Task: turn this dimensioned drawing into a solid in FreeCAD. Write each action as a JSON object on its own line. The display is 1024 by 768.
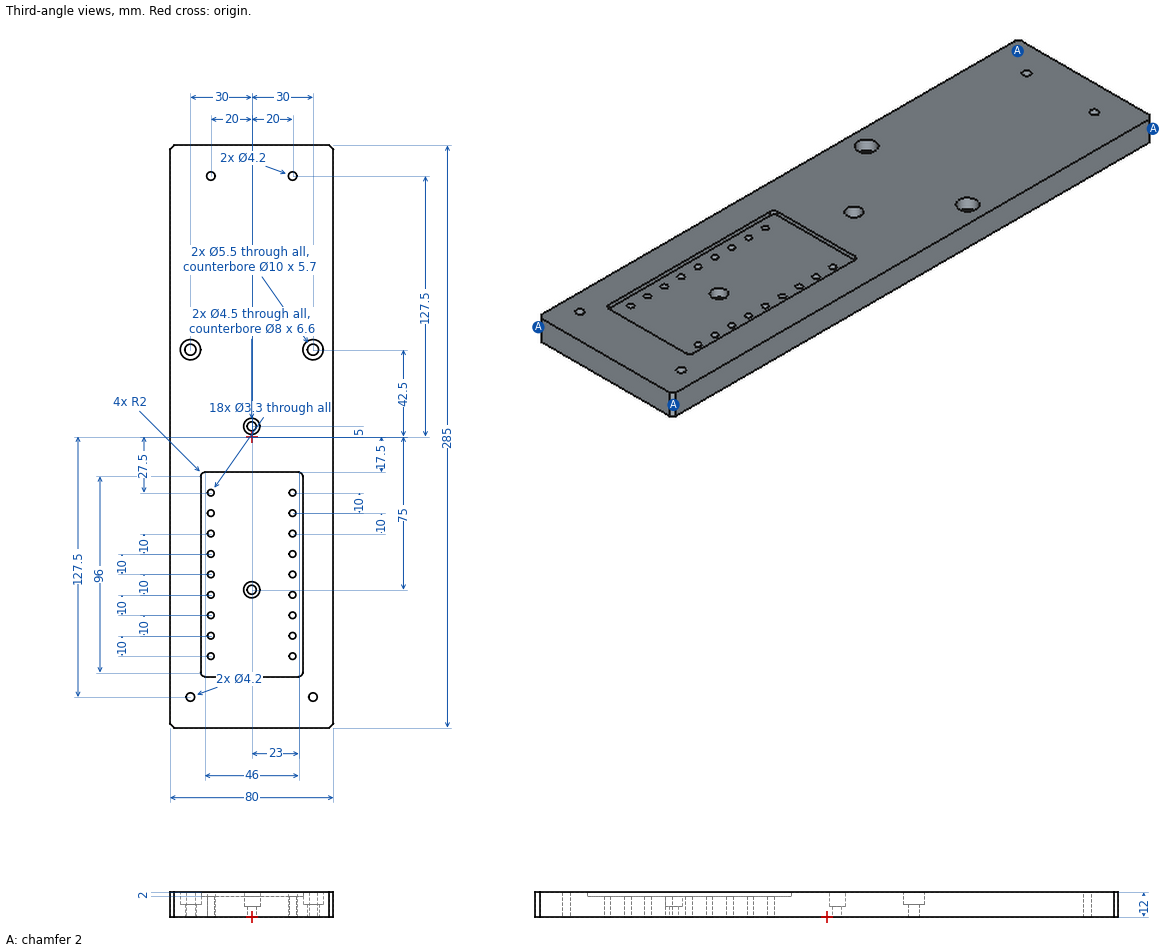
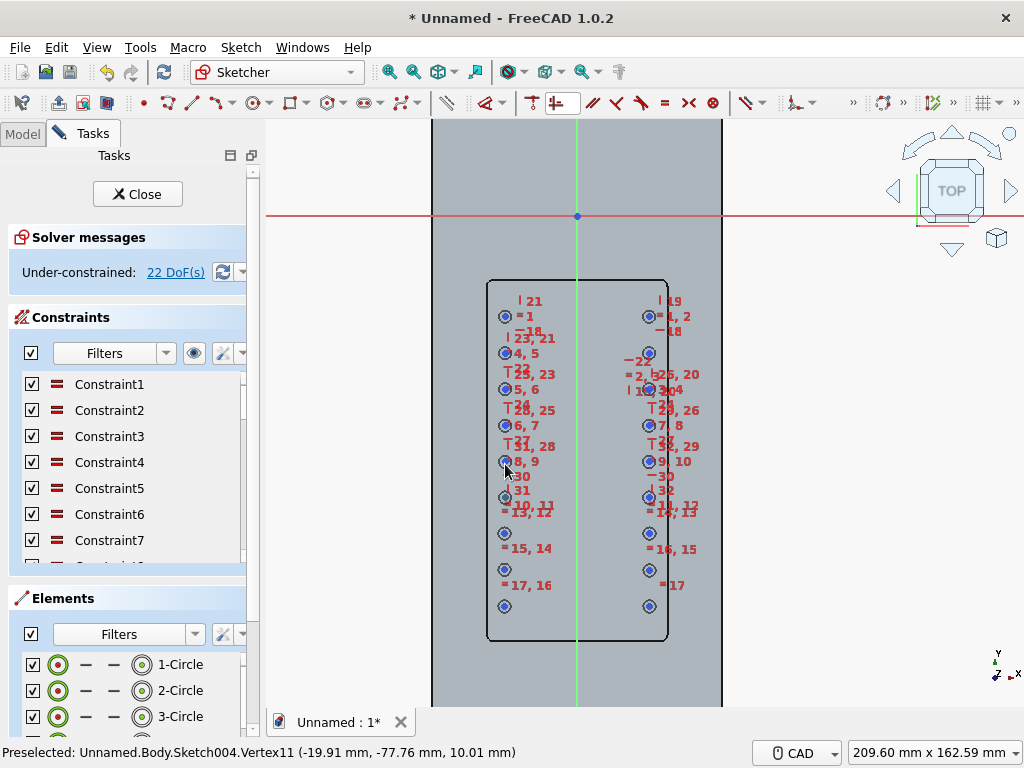
{"action": "scroll", "coordinate": [649, 498], "scroll_direction": "up", "scroll_amount": 4}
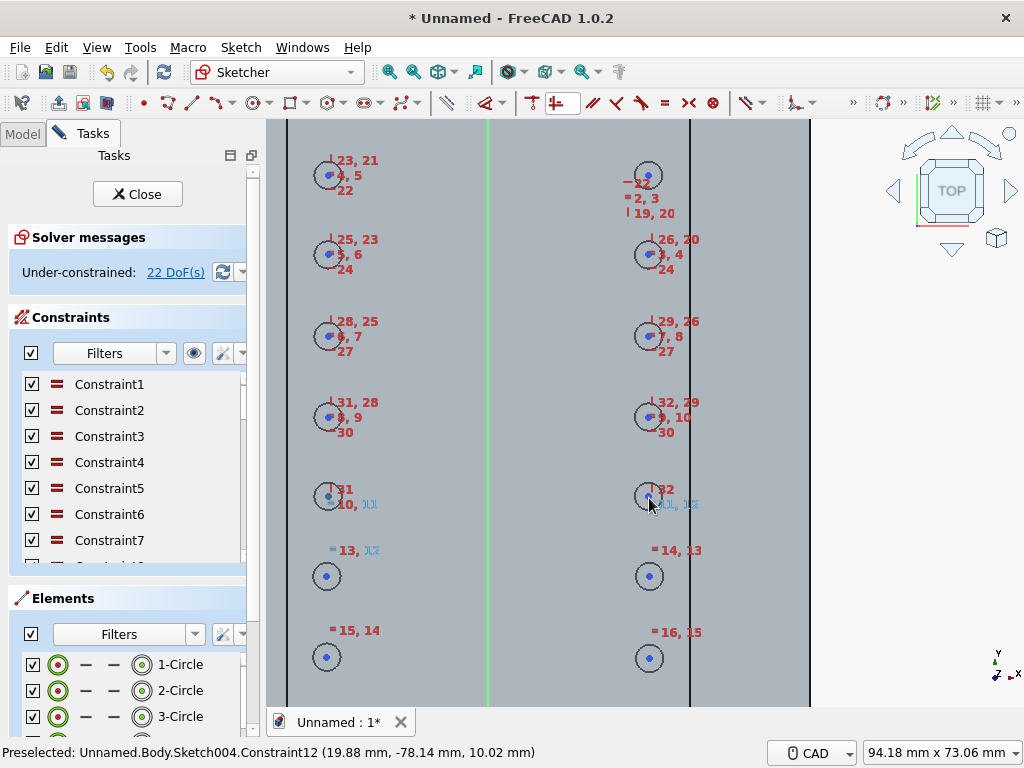
{"action": "scroll", "coordinate": [649, 496], "scroll_direction": "up", "scroll_amount": 4}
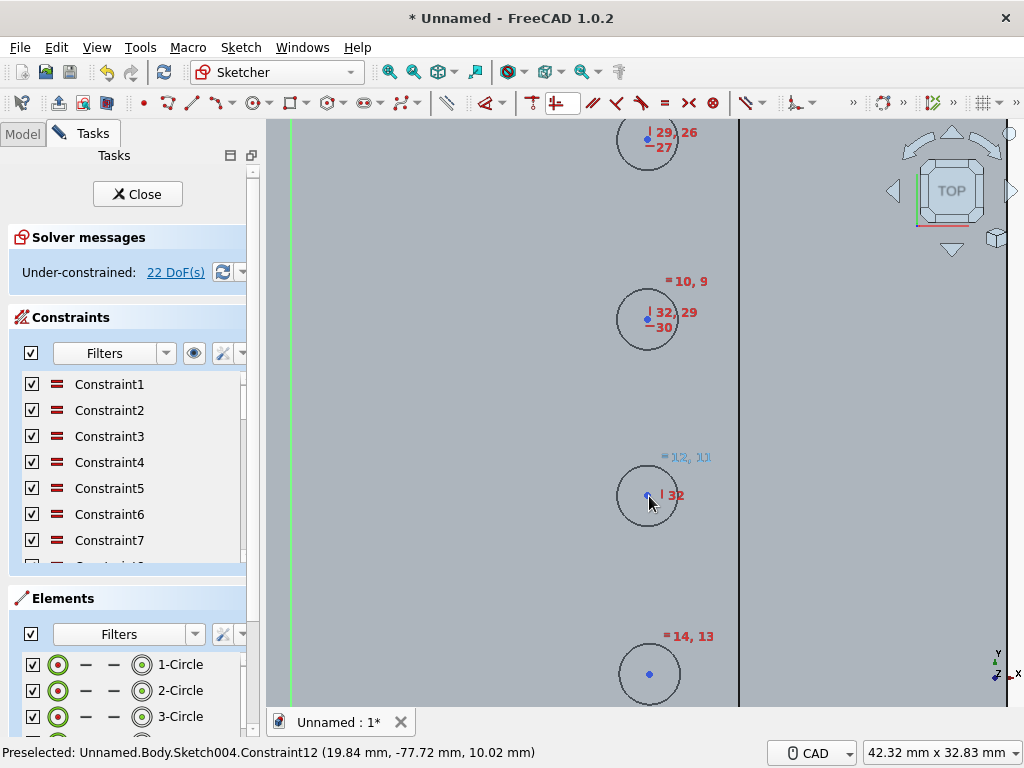
{"action": "left_click", "coordinate": [647, 496]}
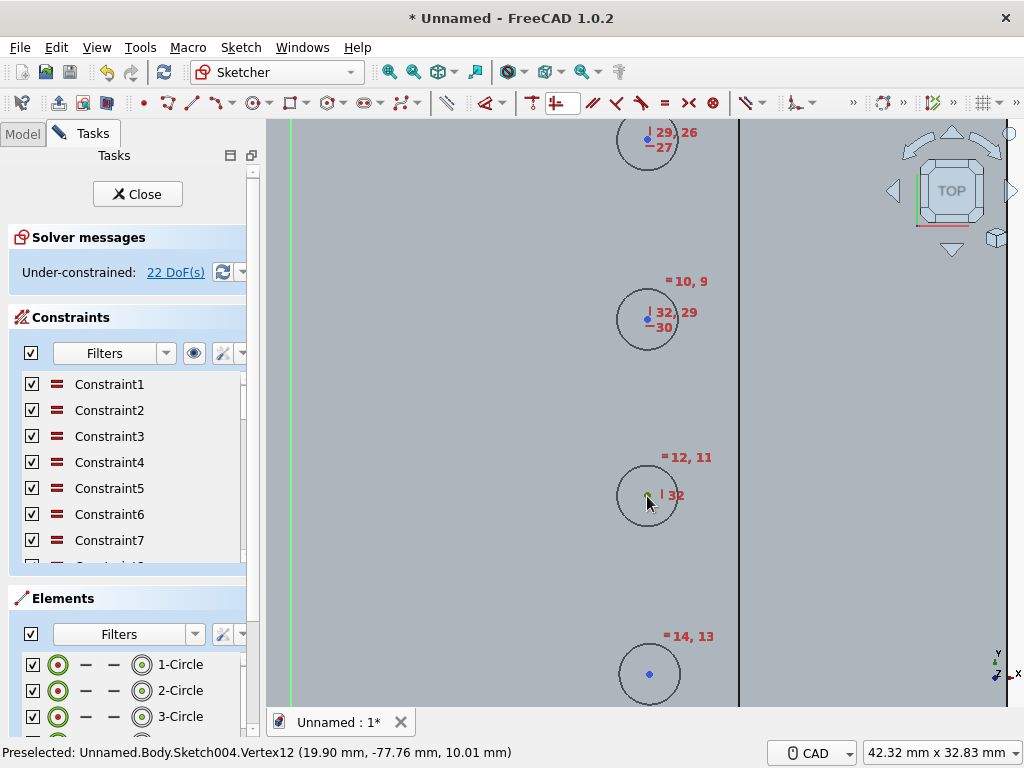
{"action": "key", "text": "h"}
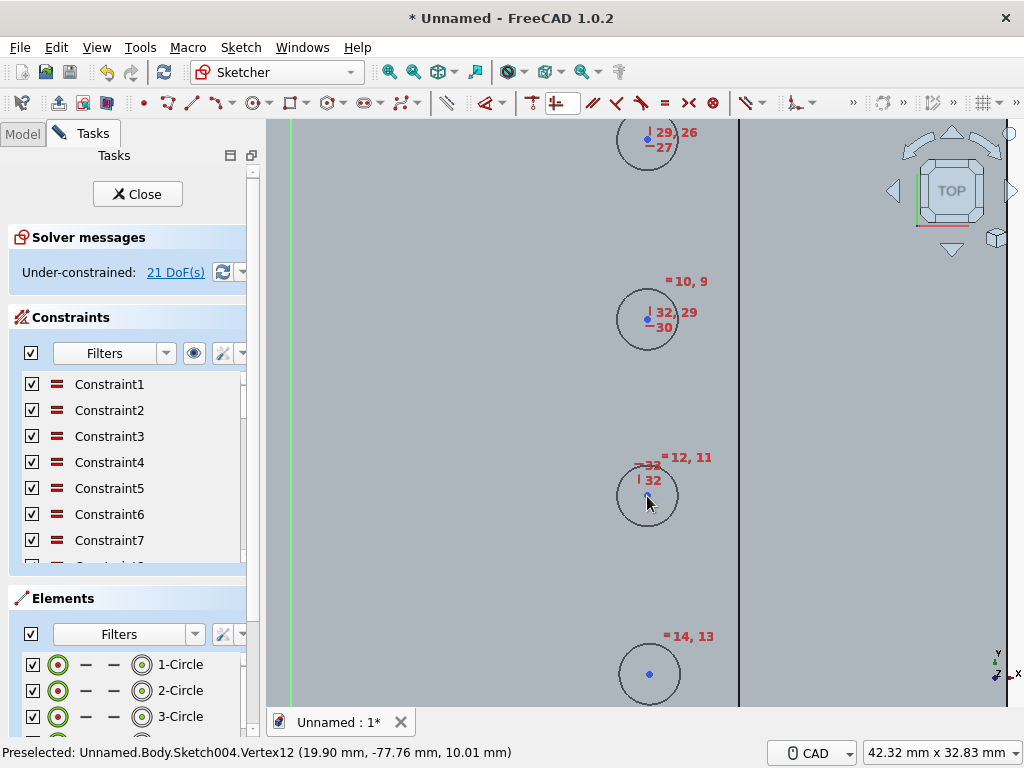
{"action": "scroll", "coordinate": [649, 497], "scroll_direction": "down", "scroll_amount": 8}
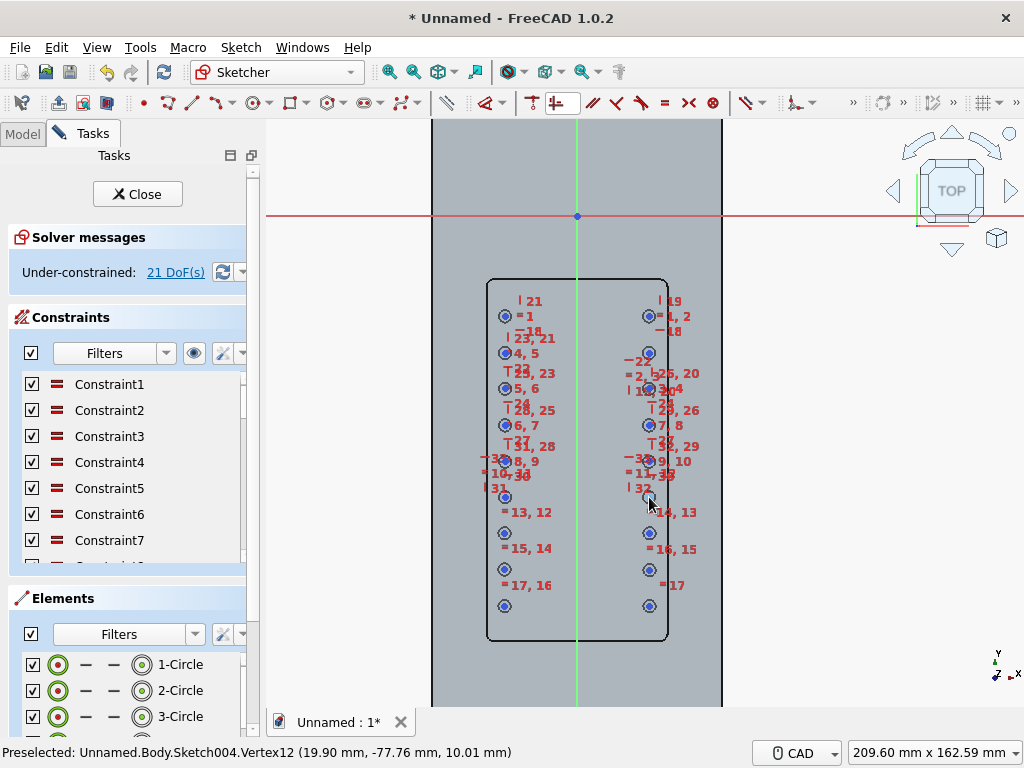
{"action": "left_click", "coordinate": [505, 497]}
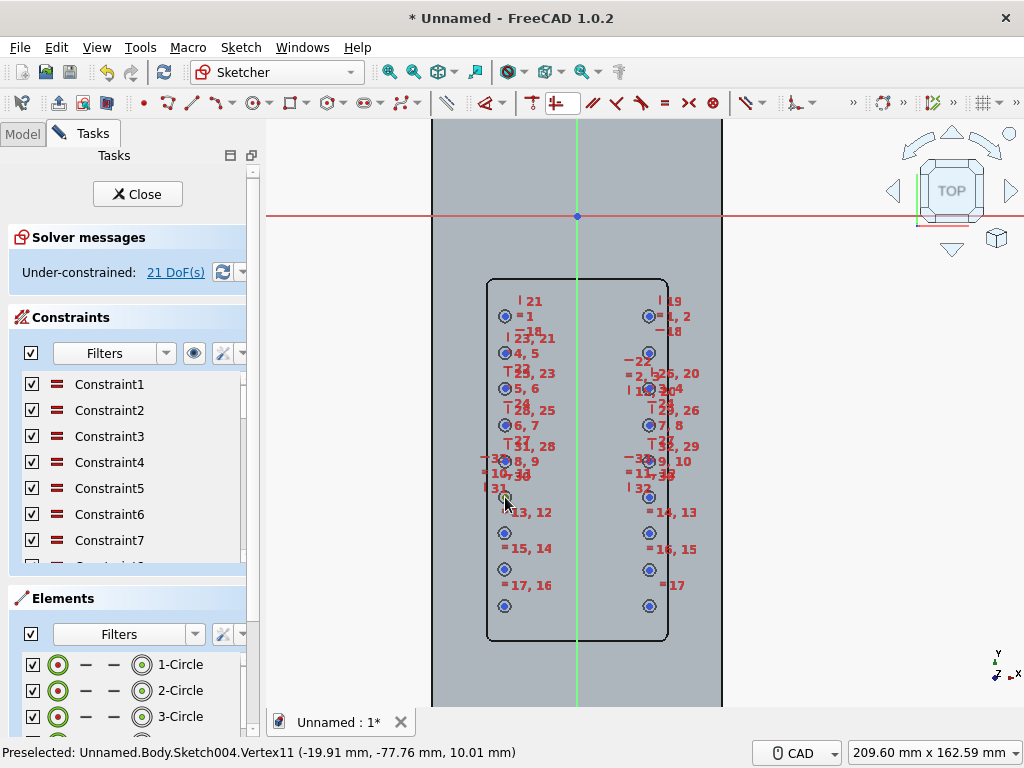
{"action": "left_click", "coordinate": [505, 533]}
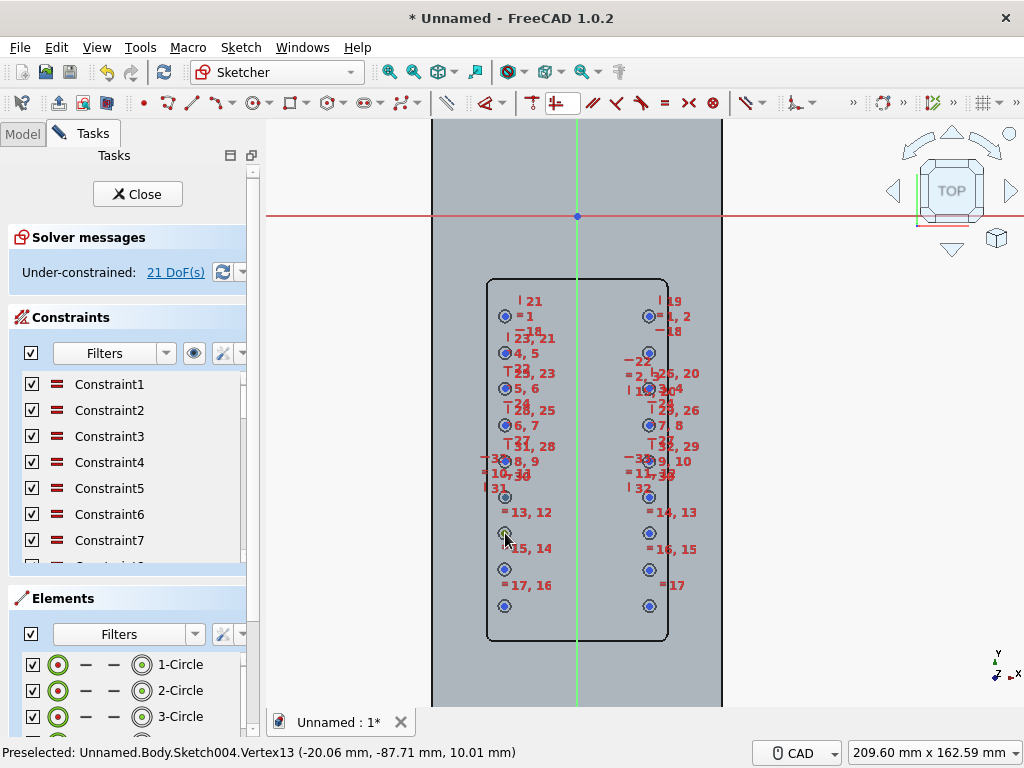
{"action": "key", "text": "v"}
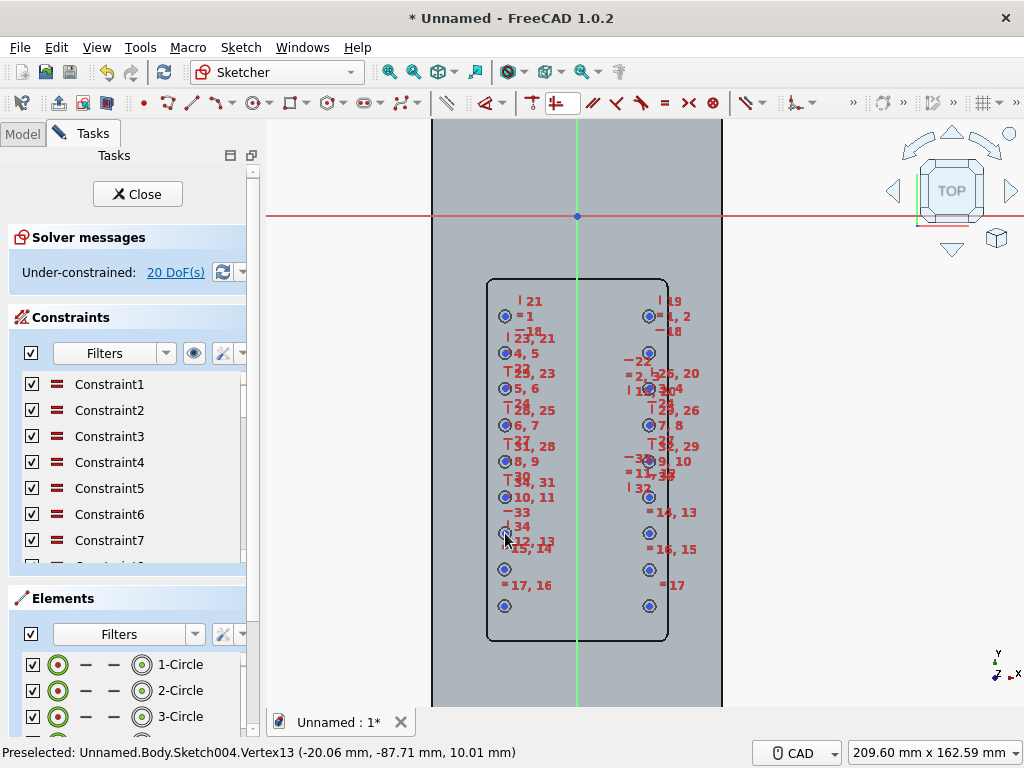
{"action": "left_click", "coordinate": [649, 497]}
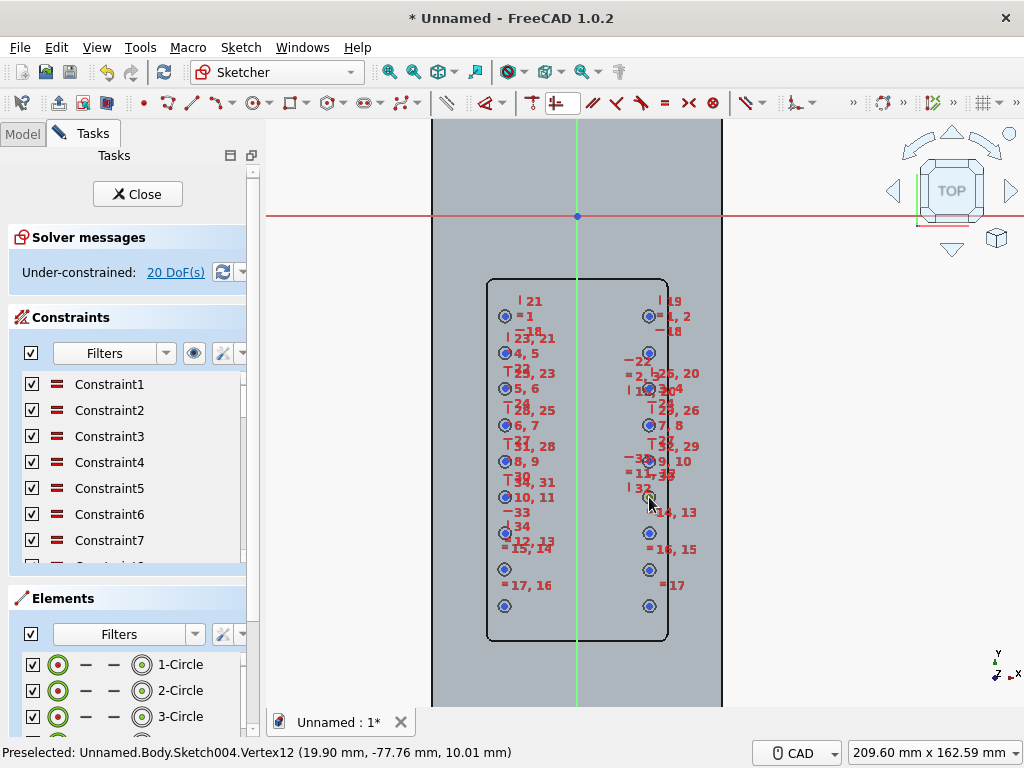
{"action": "left_click", "coordinate": [650, 533]}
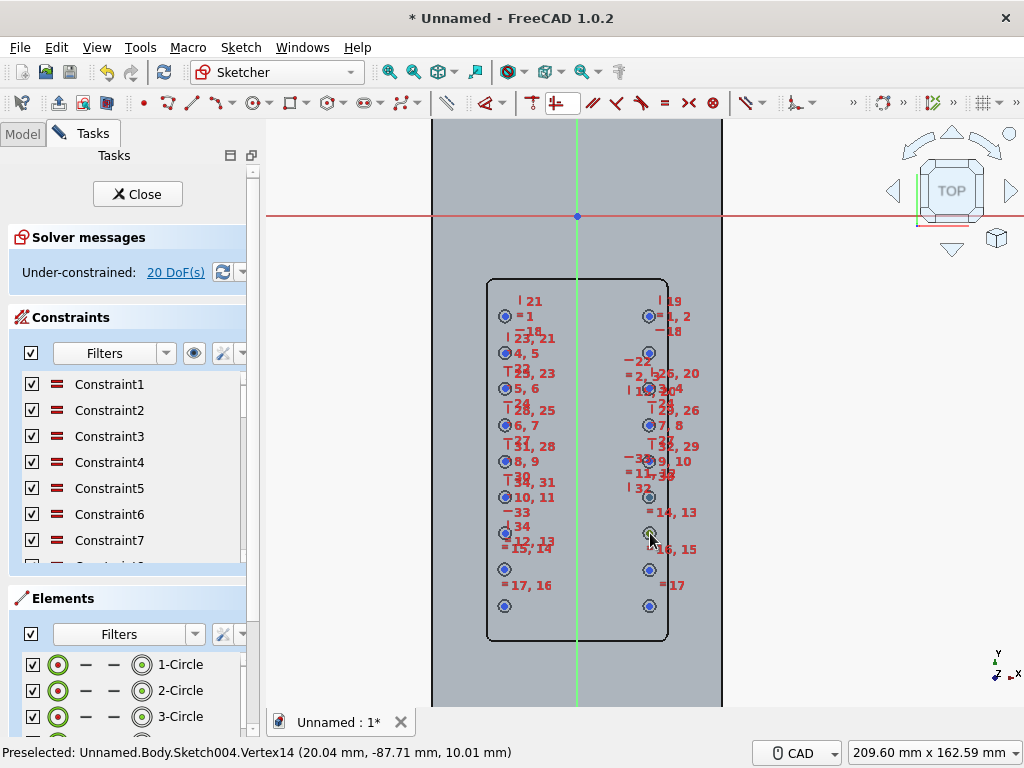
{"action": "key", "text": "v"}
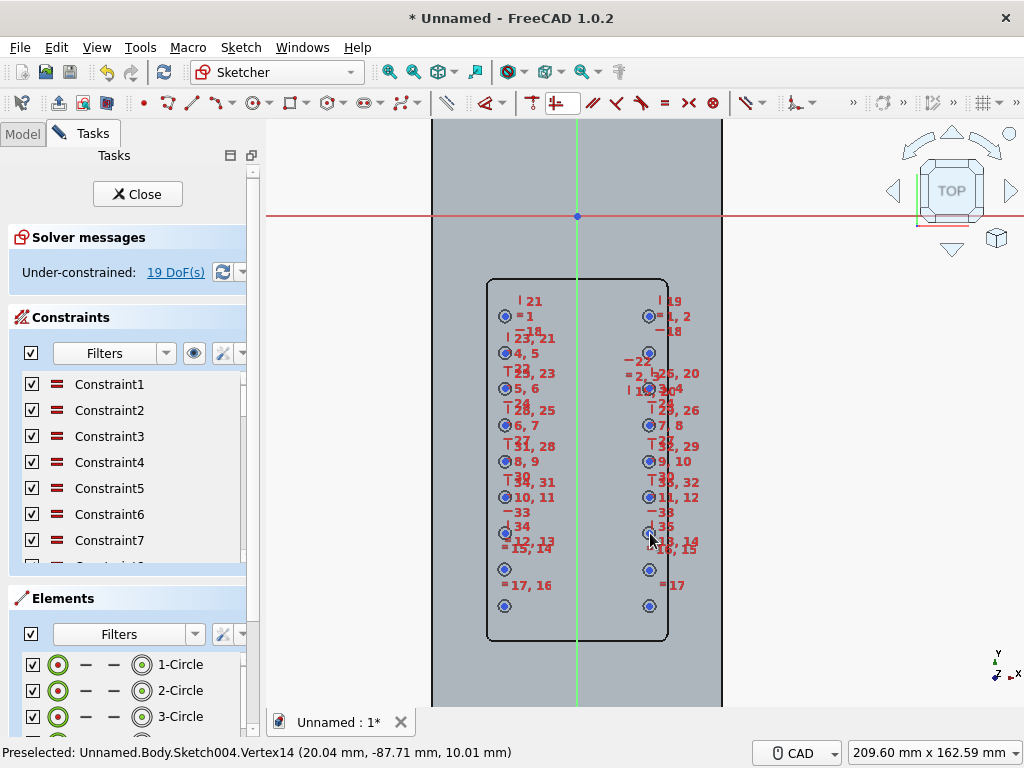
{"action": "scroll", "coordinate": [505, 533], "scroll_direction": "up", "scroll_amount": 4}